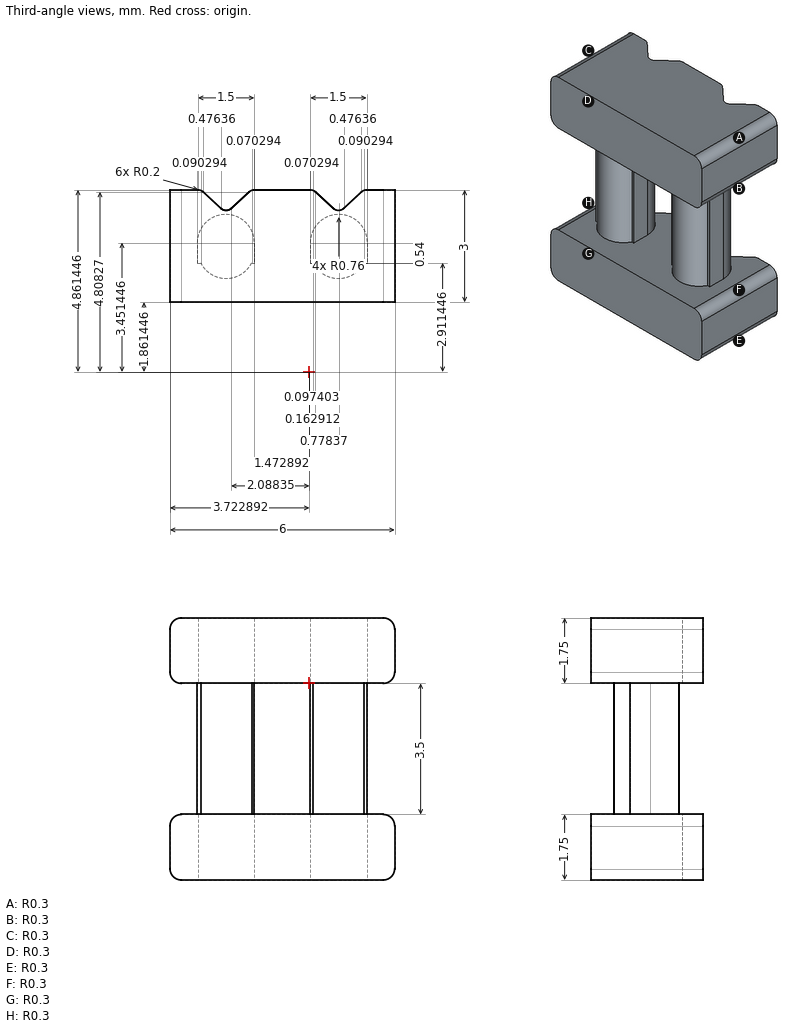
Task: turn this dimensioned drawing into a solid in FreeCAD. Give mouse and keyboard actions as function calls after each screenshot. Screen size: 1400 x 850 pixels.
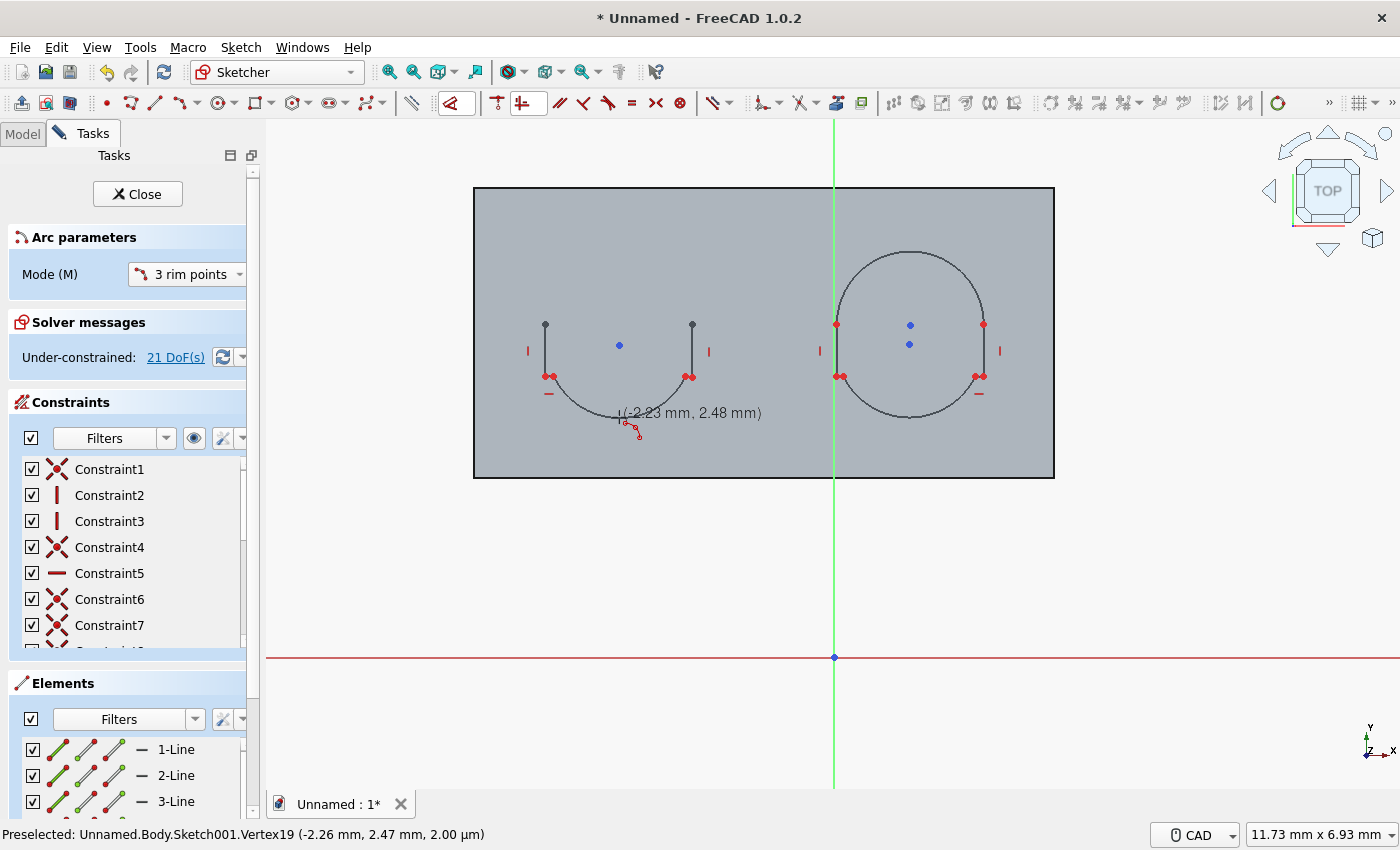
click(545, 324)
click(692, 325)
click(618, 251)
key(Escape)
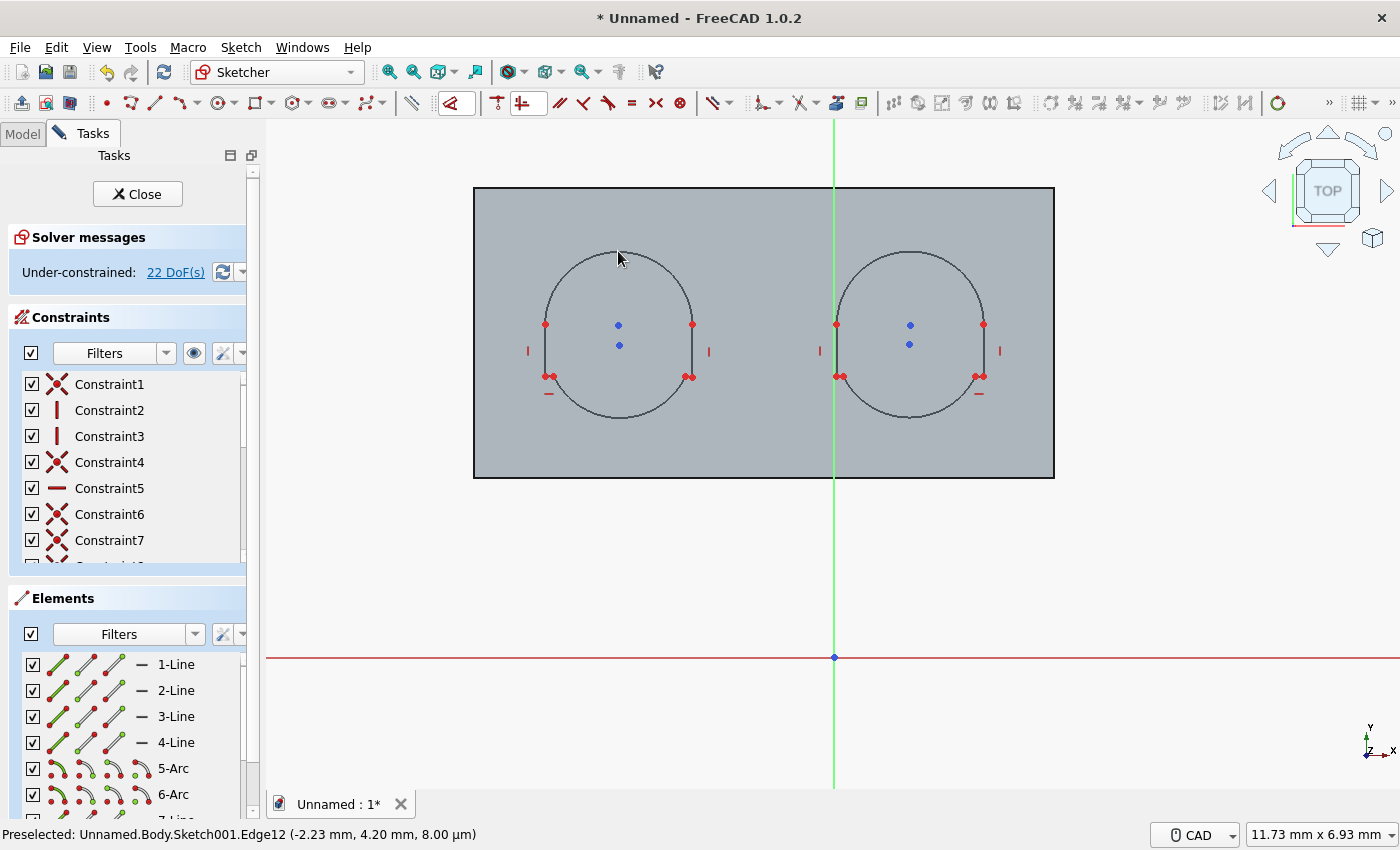
click(837, 361)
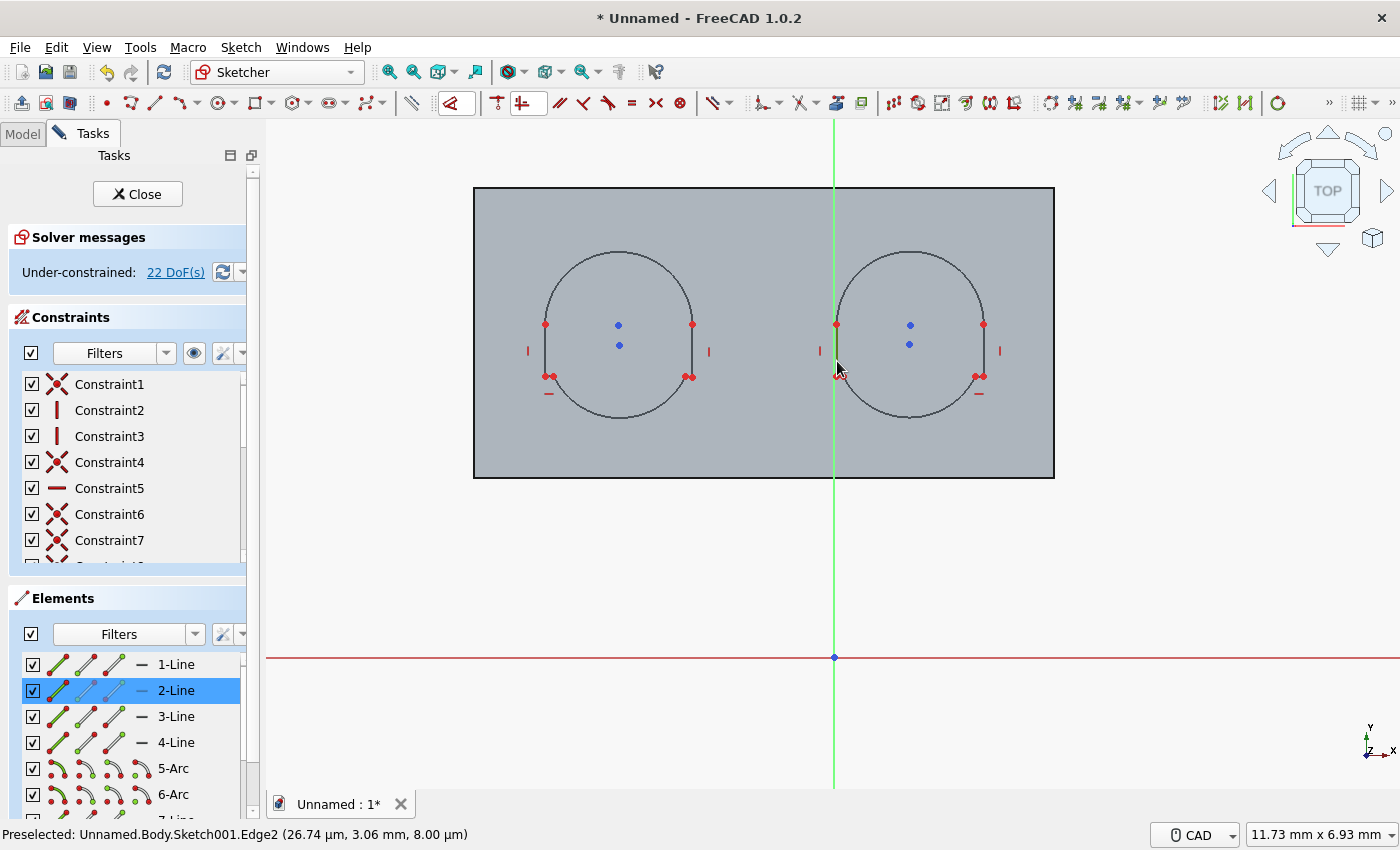
click(954, 266)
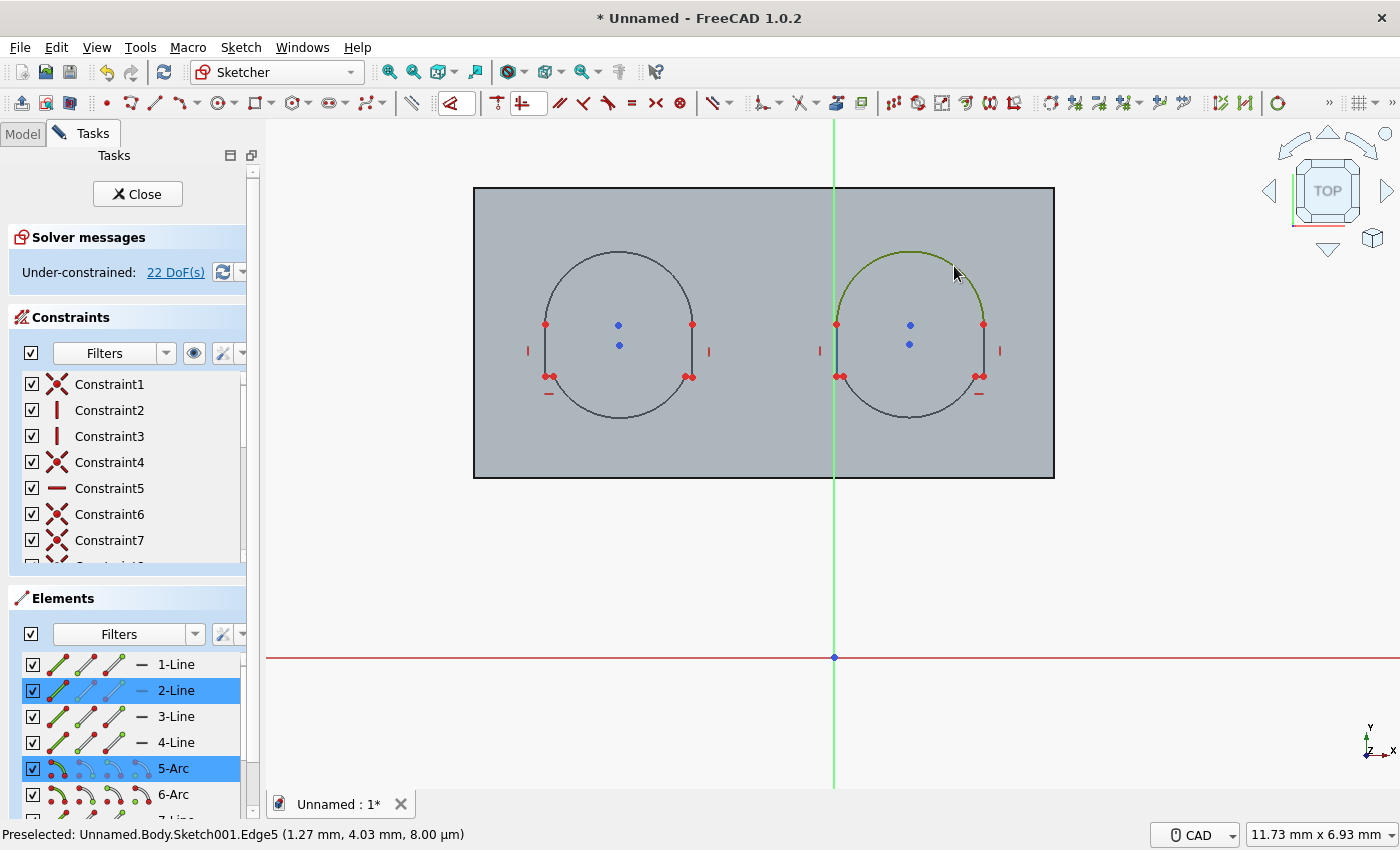
click(608, 104)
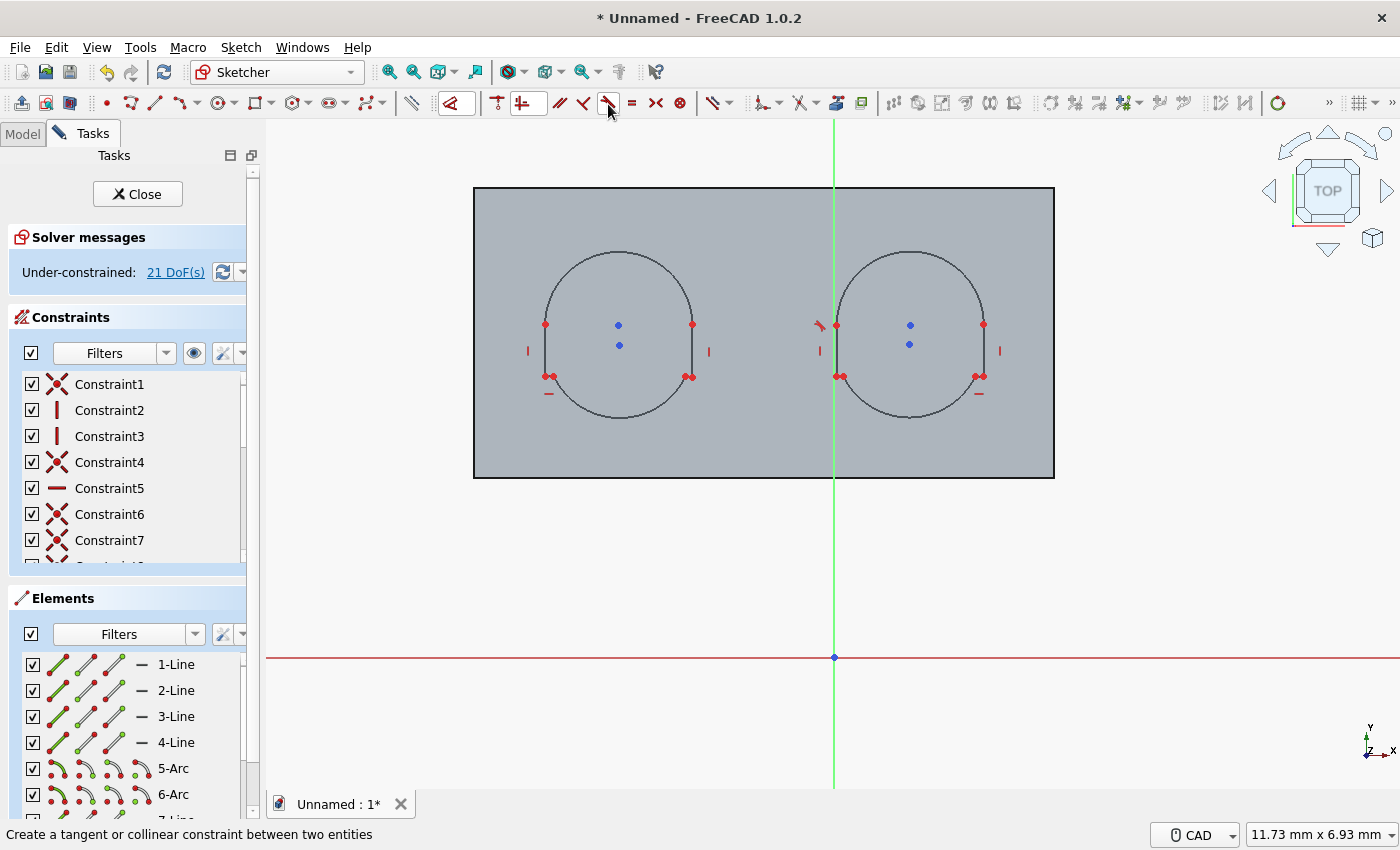
click(984, 341)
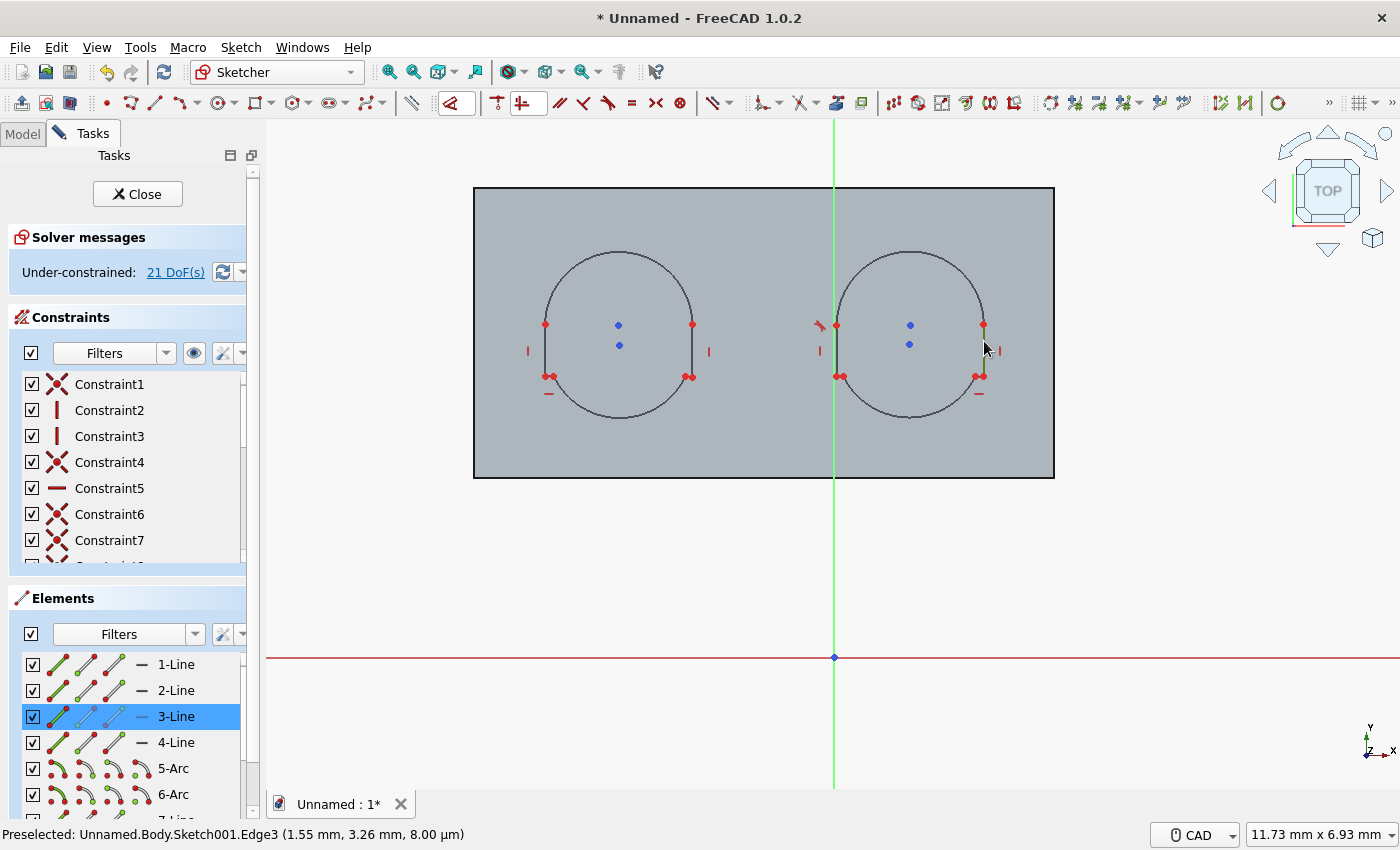
click(953, 266)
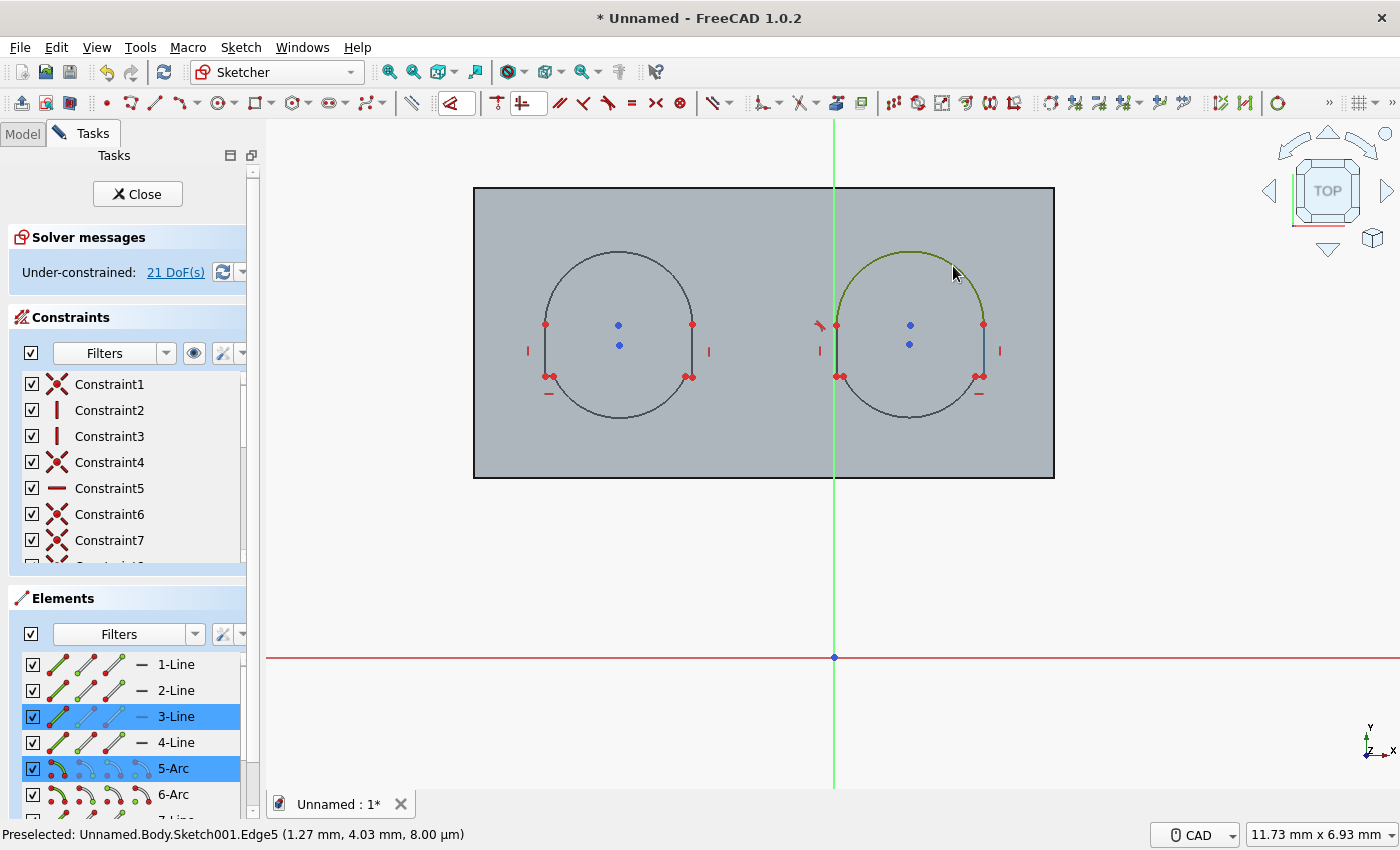
click(608, 104)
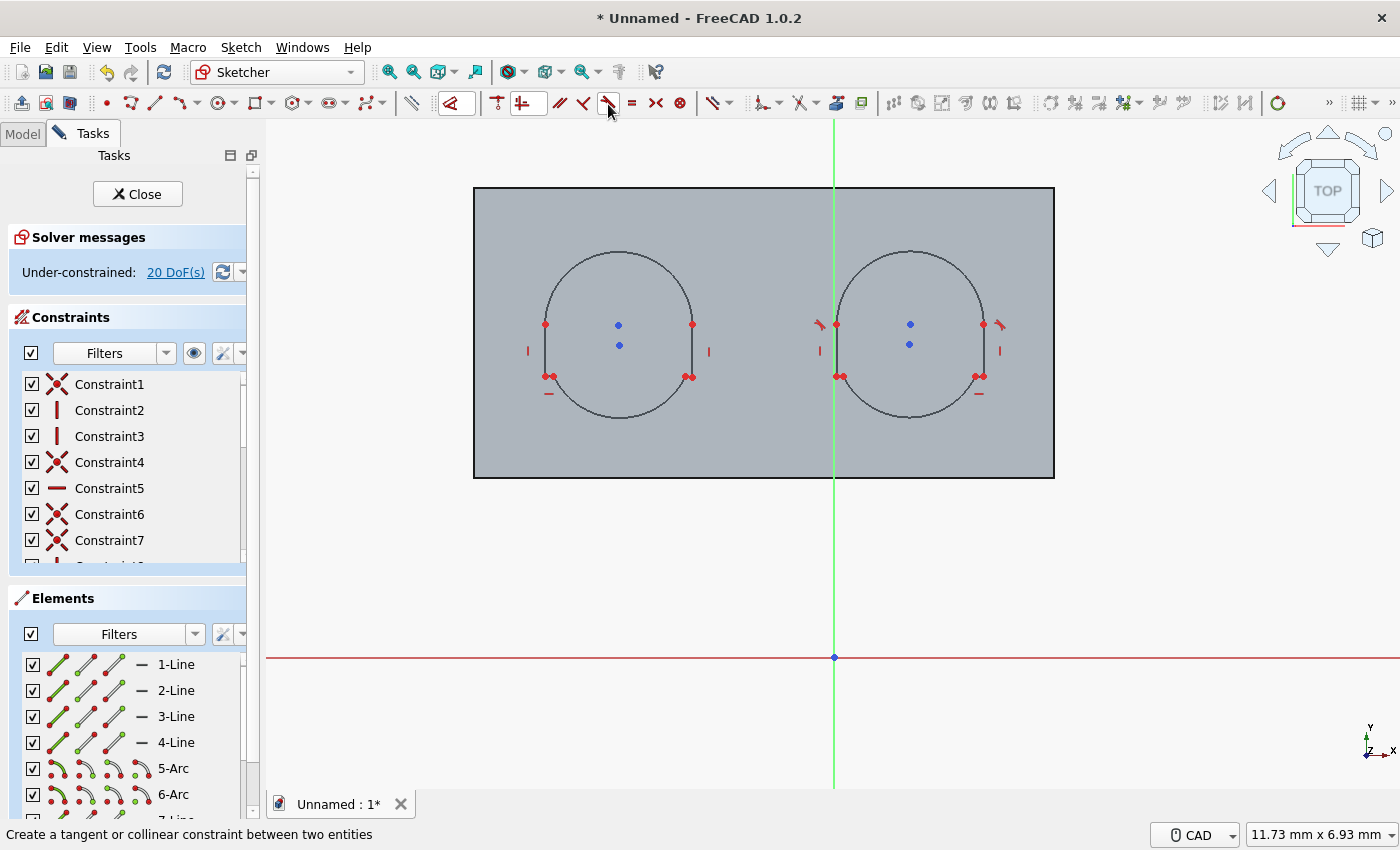
click(692, 340)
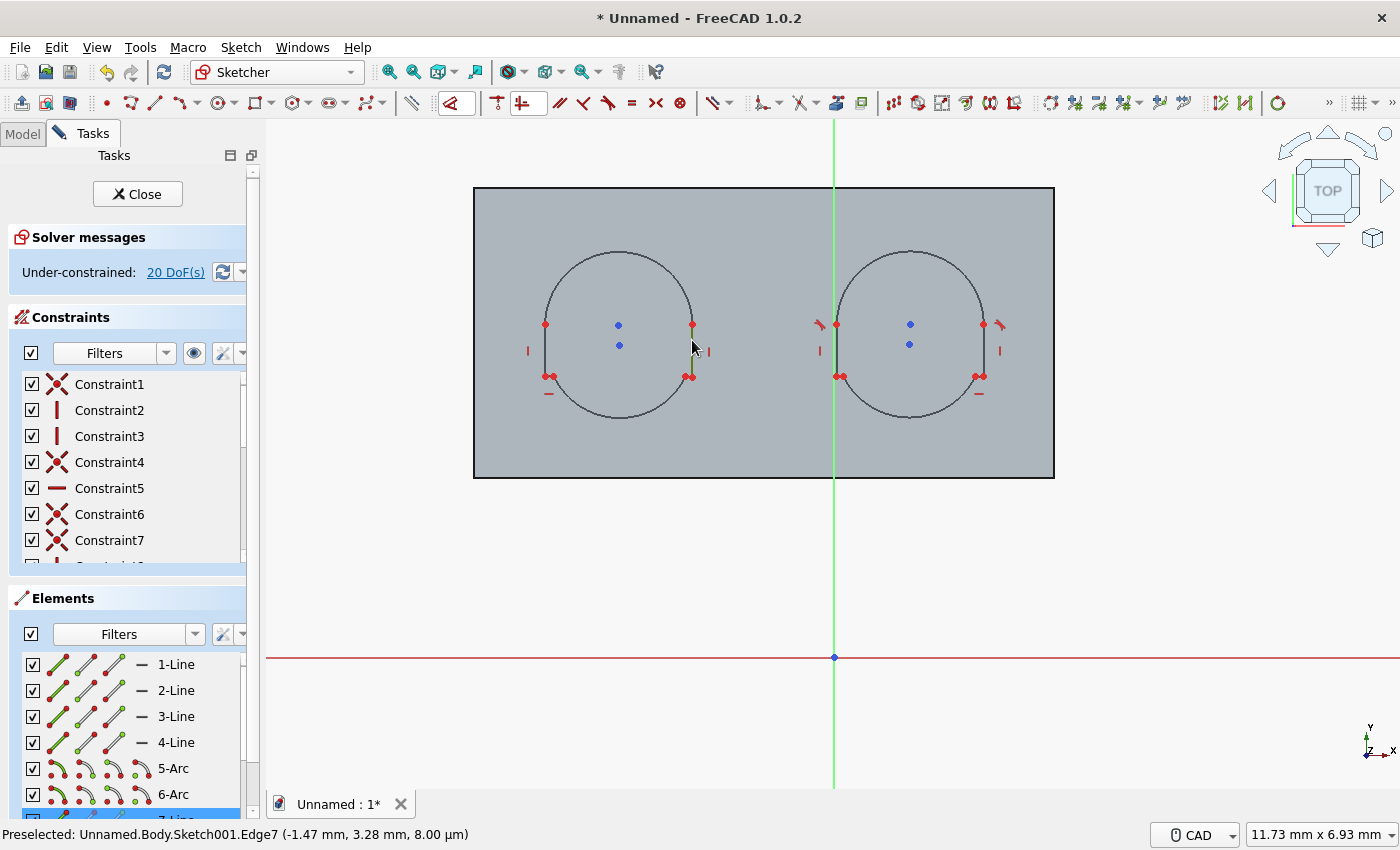
click(662, 266)